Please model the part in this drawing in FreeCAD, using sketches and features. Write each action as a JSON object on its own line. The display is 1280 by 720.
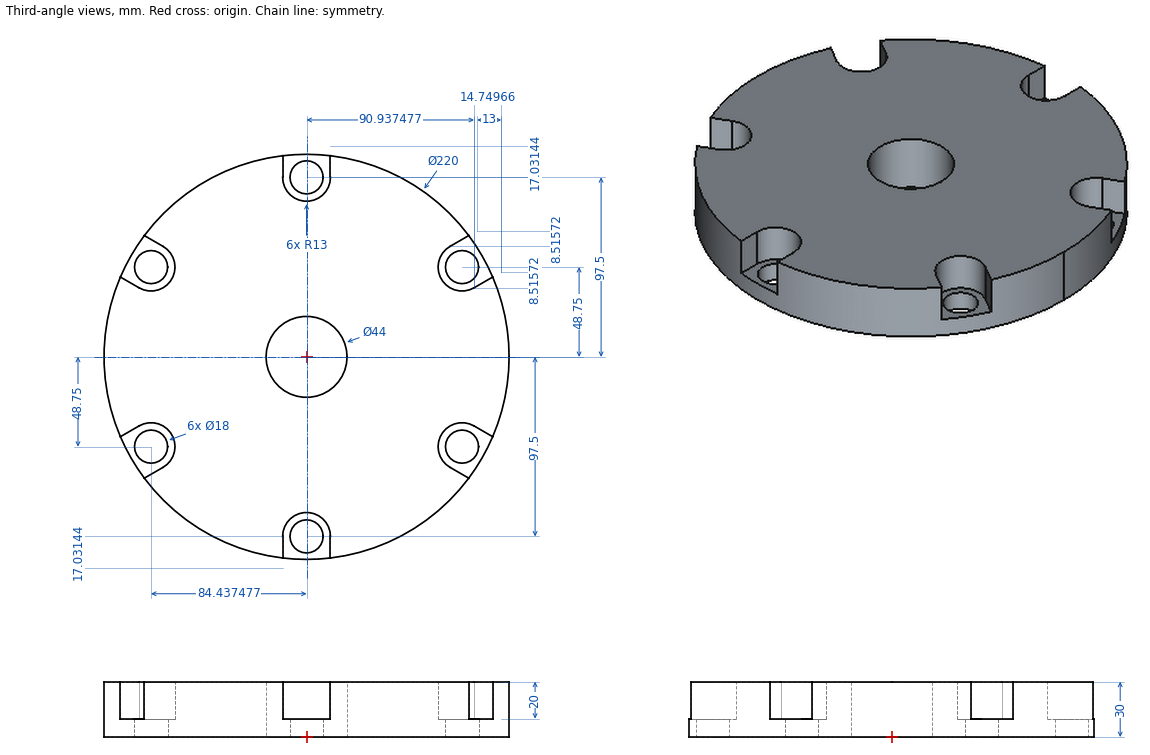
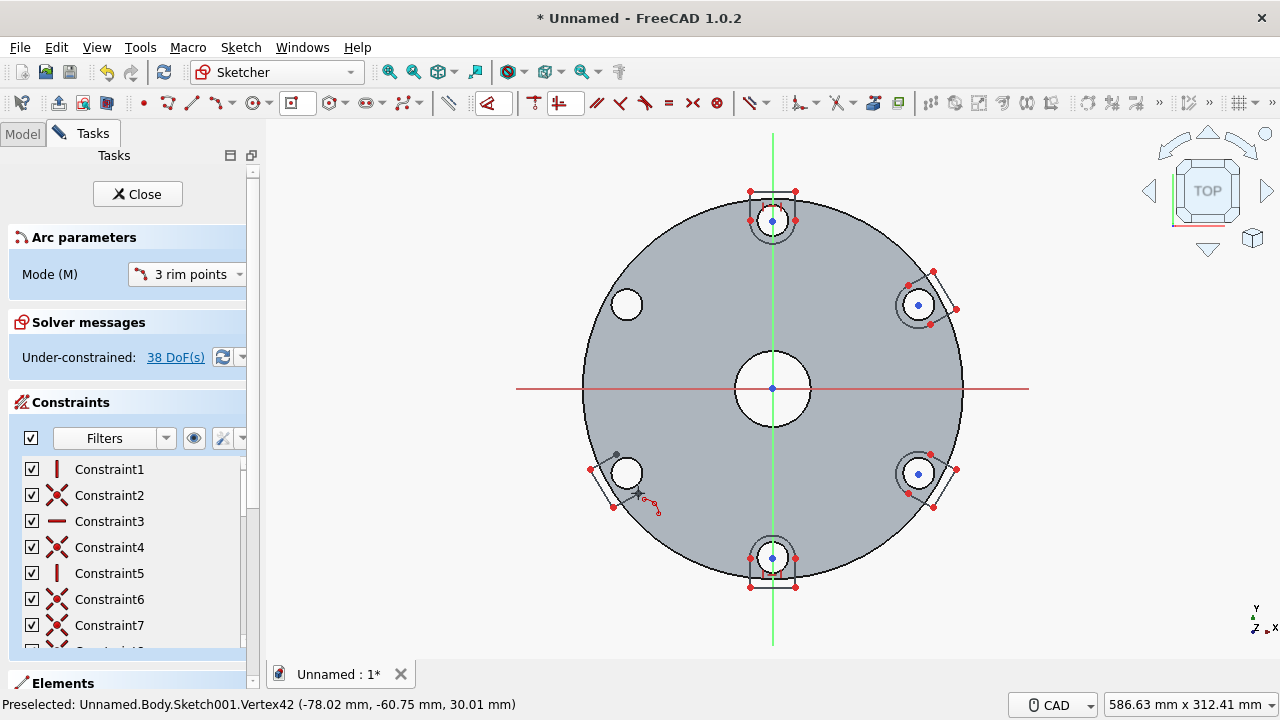
{"action": "left_click", "coordinate": [638, 494]}
{"action": "left_click", "coordinate": [616, 455]}
{"action": "left_click", "coordinate": [646, 462]}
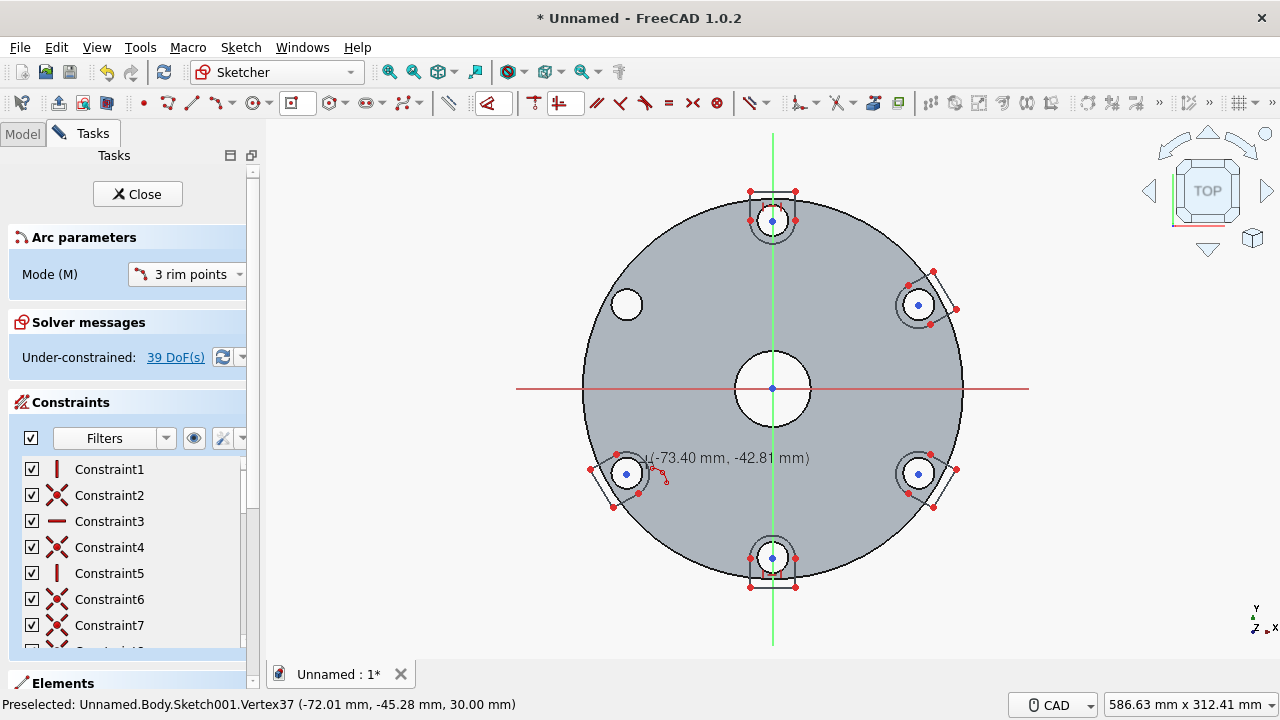
{"action": "left_click", "coordinate": [168, 104]}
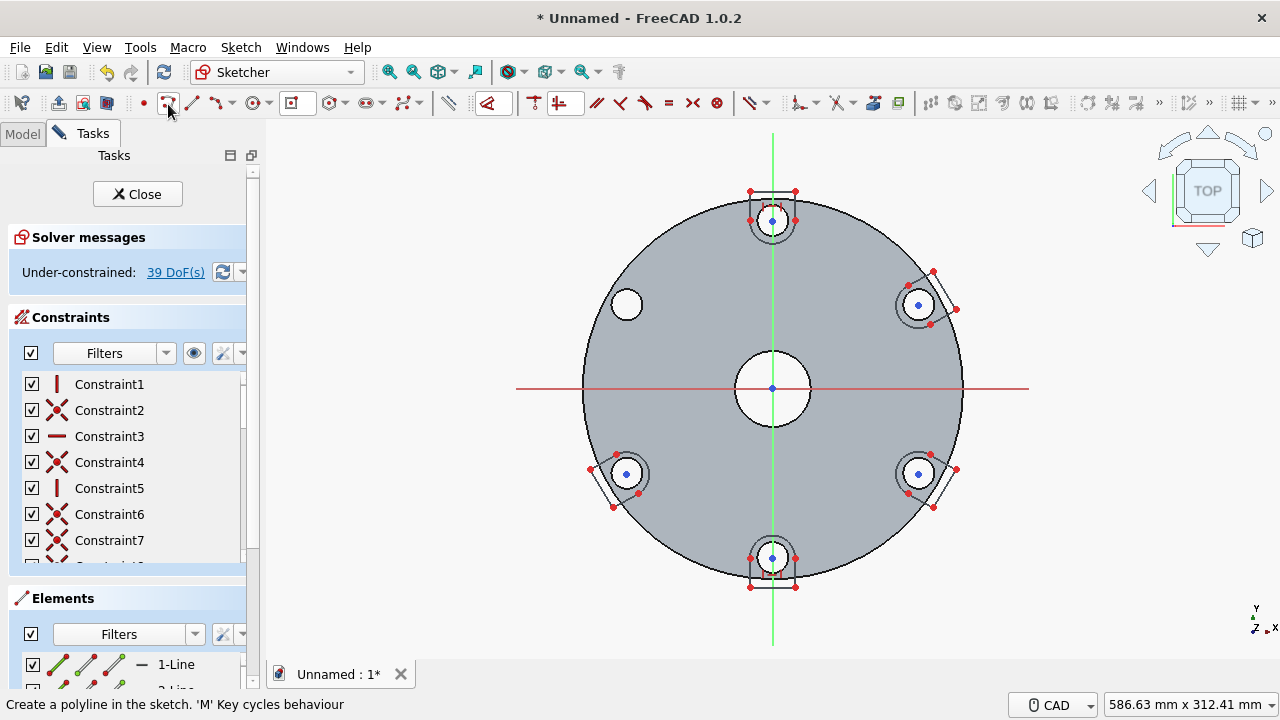
{"action": "left_click", "coordinate": [638, 285]}
{"action": "left_click", "coordinate": [613, 271]}
{"action": "left_click", "coordinate": [590, 309]}
{"action": "left_click", "coordinate": [616, 324]}
{"action": "right_click", "coordinate": [616, 324]}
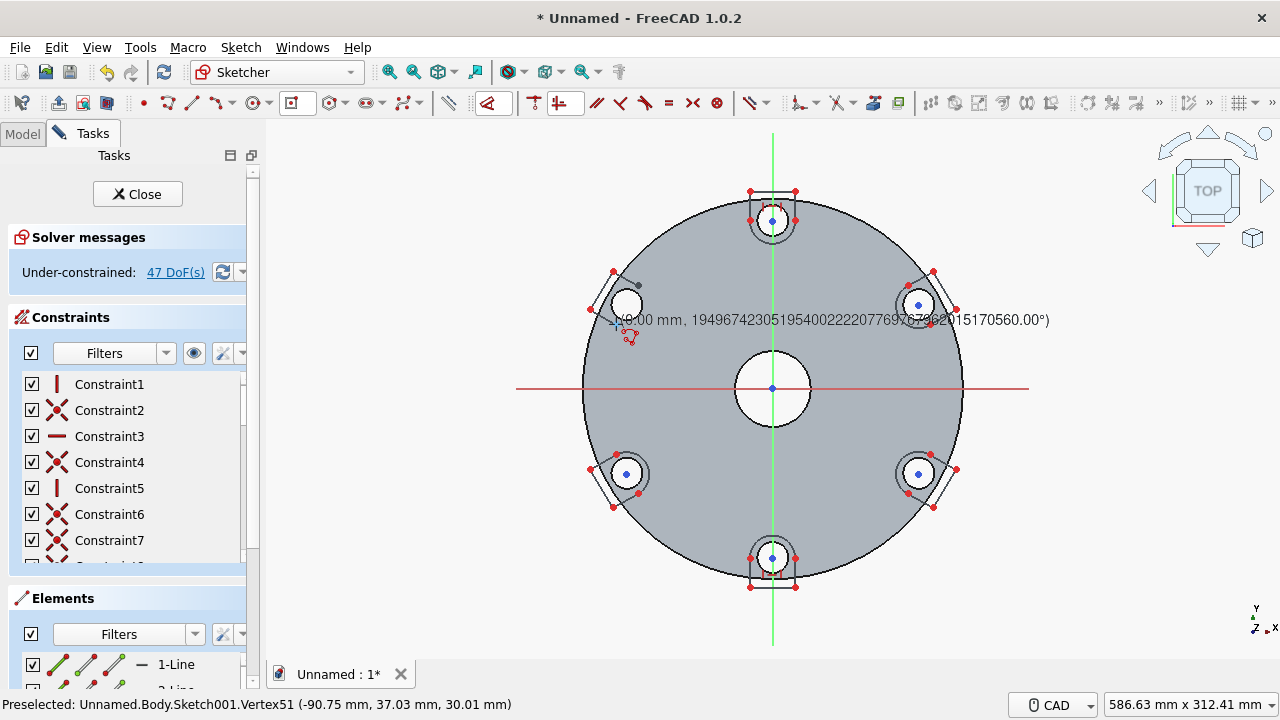
{"action": "key", "text": "g 3 a"}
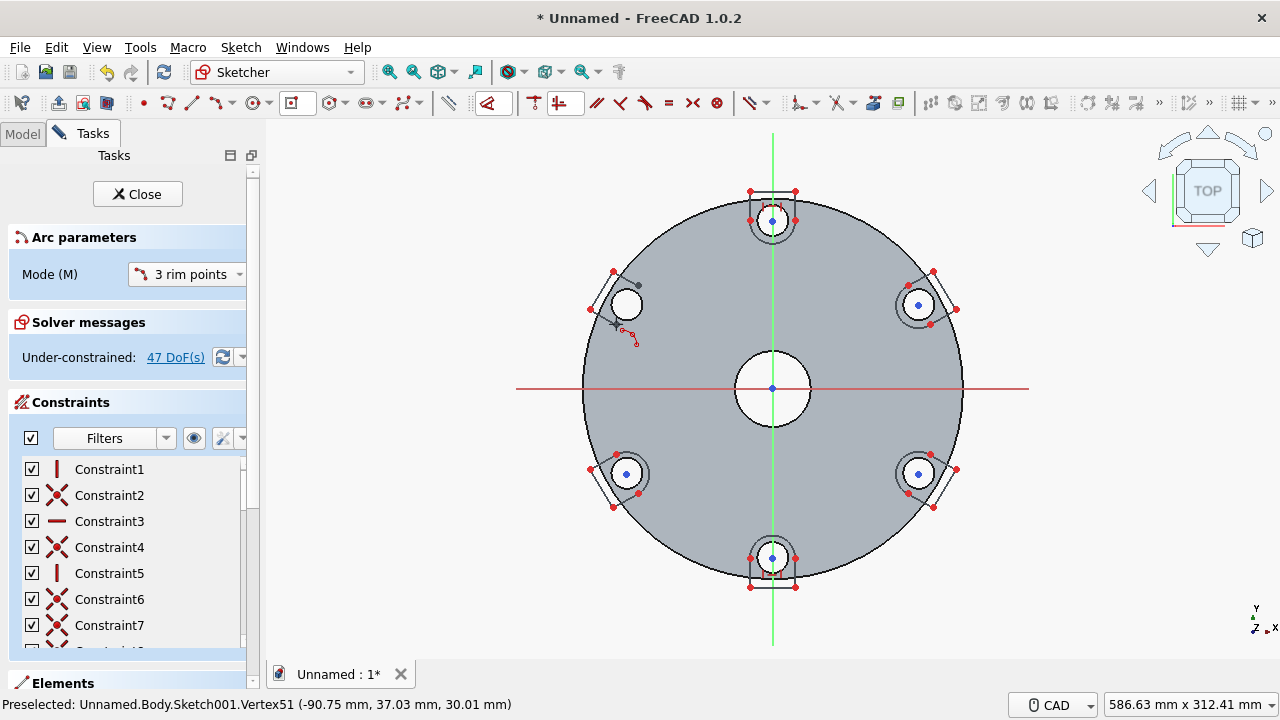
{"action": "left_click", "coordinate": [616, 325]}
{"action": "left_click", "coordinate": [638, 286]}
{"action": "left_click", "coordinate": [646, 316]}
{"action": "key", "text": "Escape"}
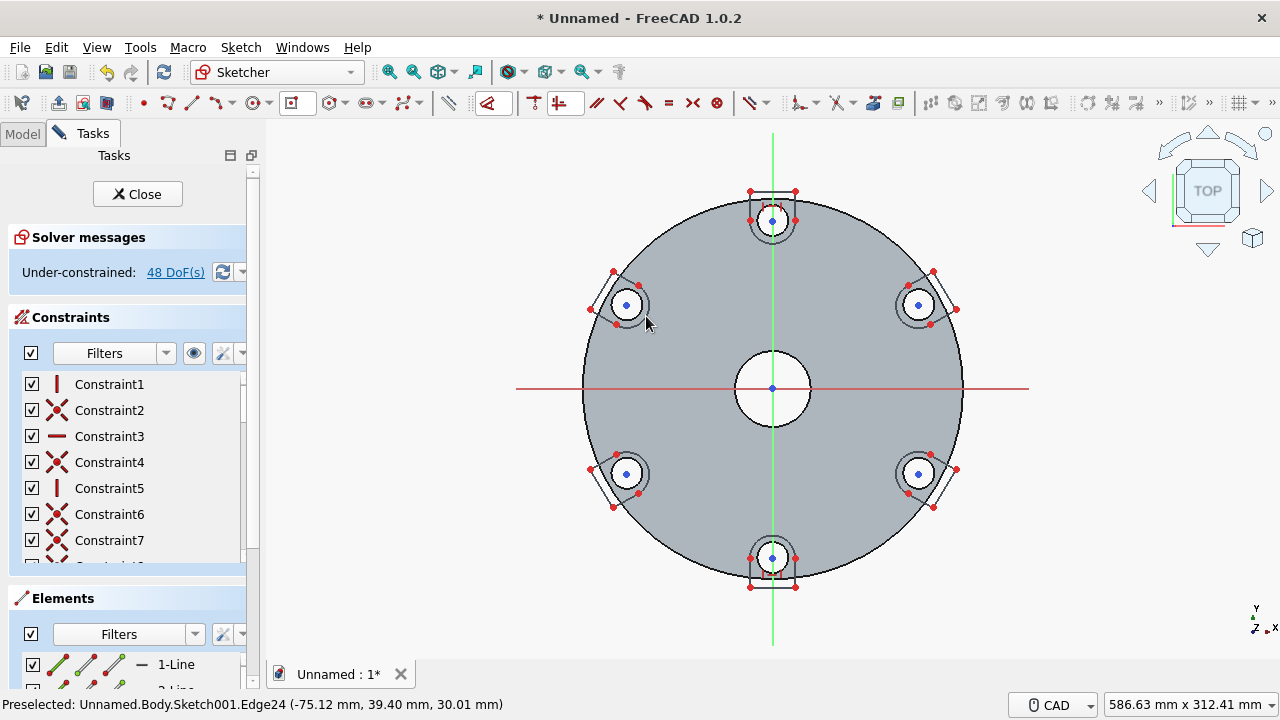
{"action": "left_click", "coordinate": [795, 209]}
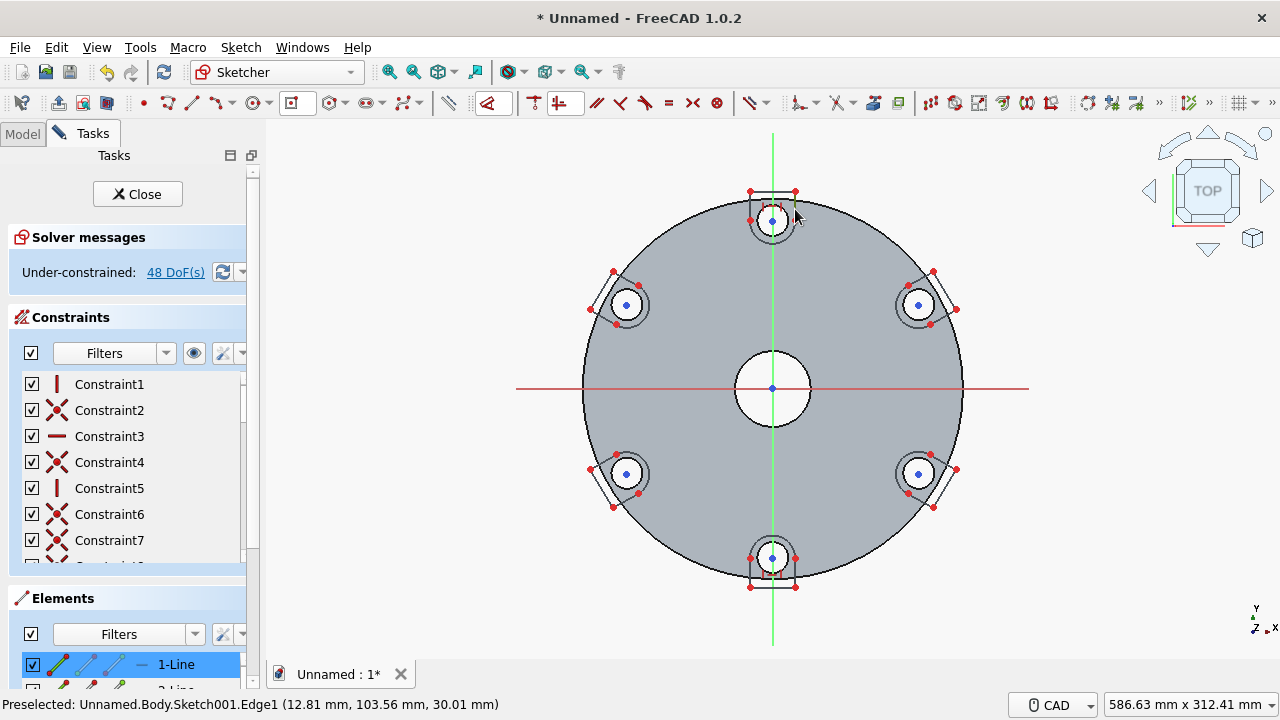
{"action": "left_click", "coordinate": [759, 239]}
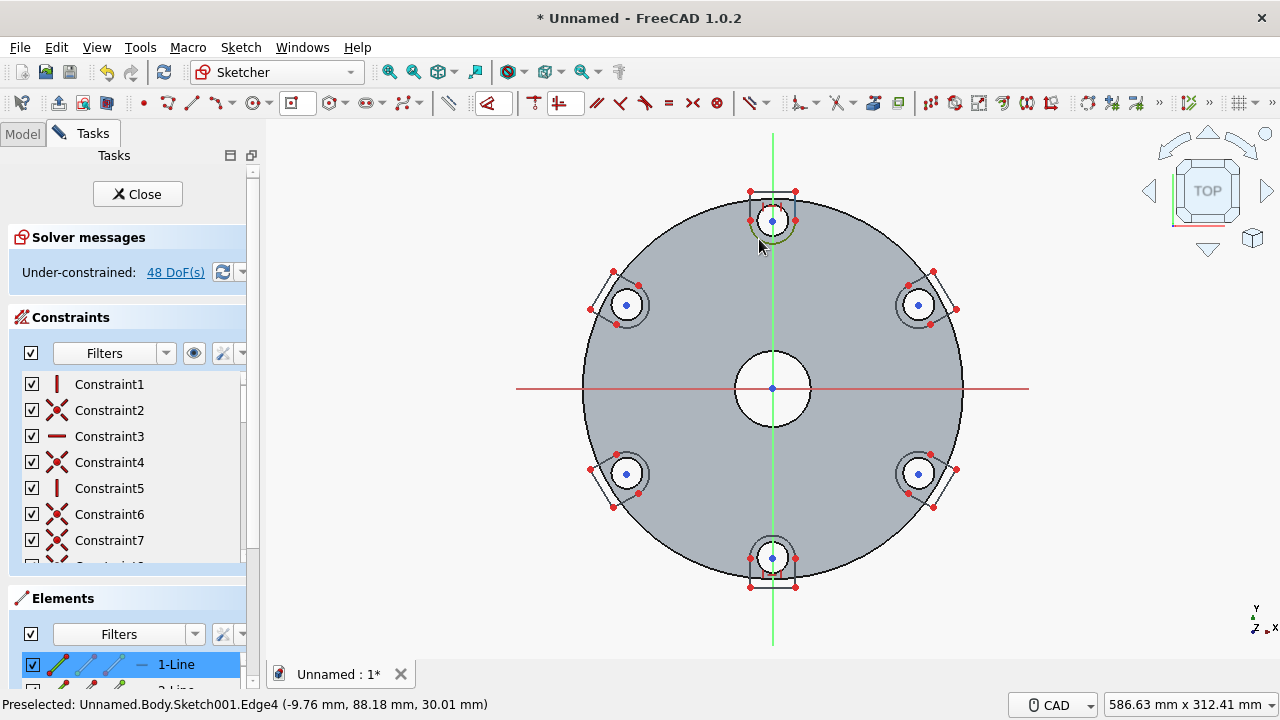
{"action": "left_click", "coordinate": [646, 104]}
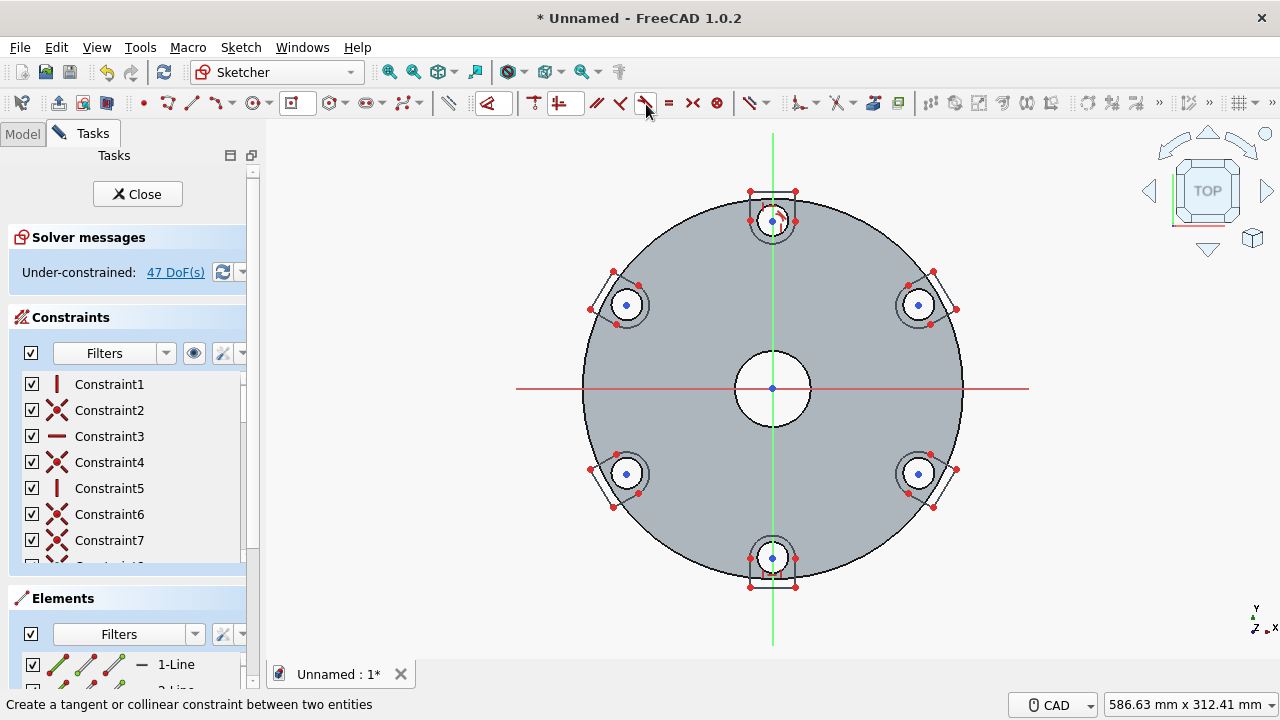
{"action": "left_click", "coordinate": [750, 204]}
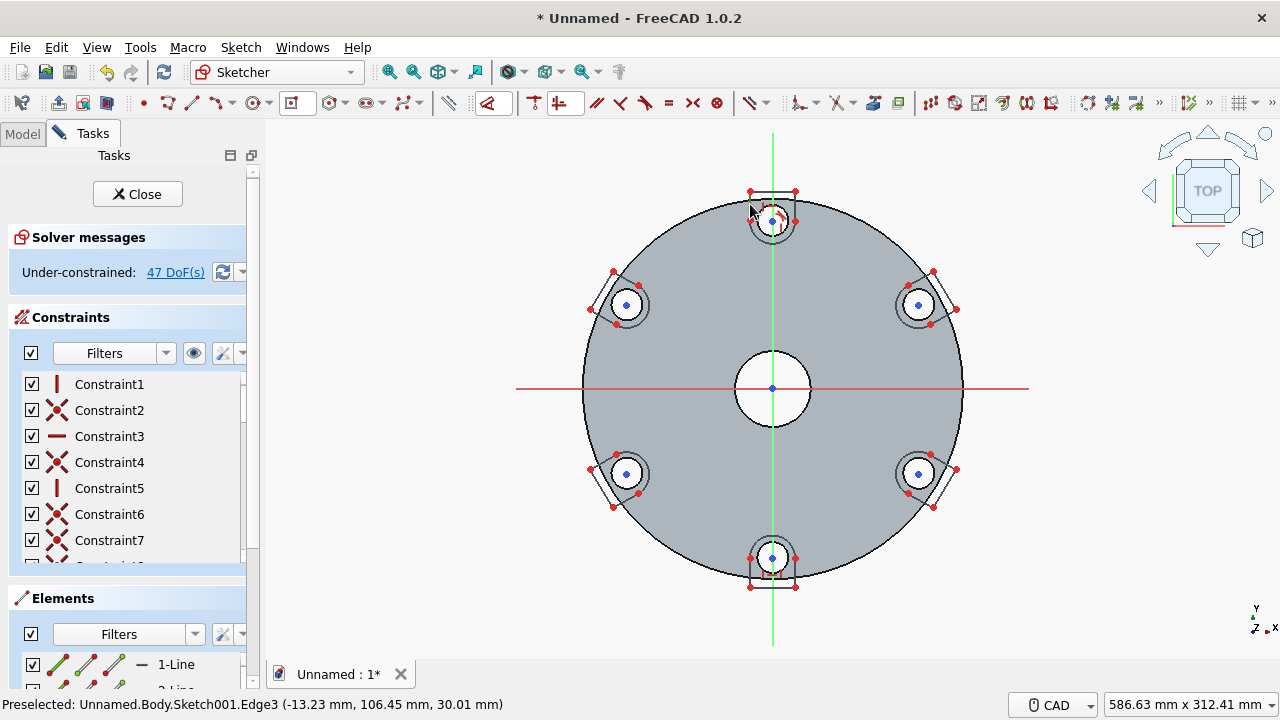
{"action": "left_click", "coordinate": [759, 239]}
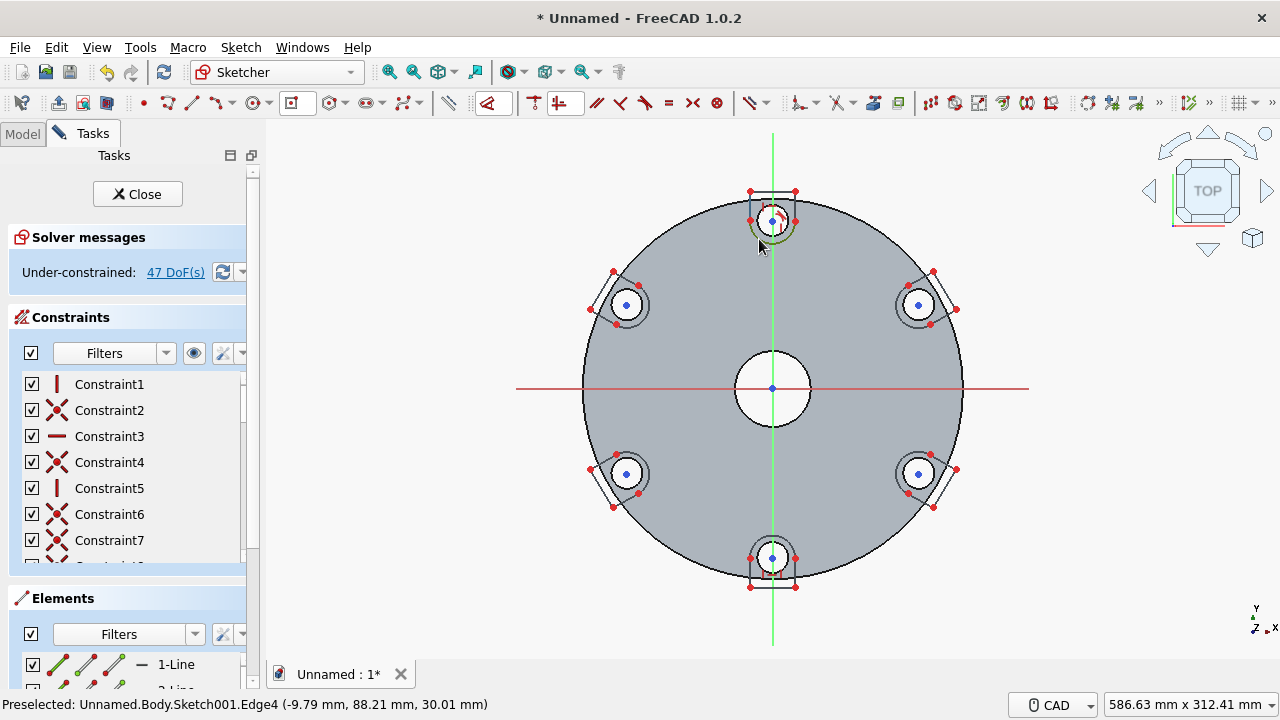
{"action": "left_click", "coordinate": [646, 104]}